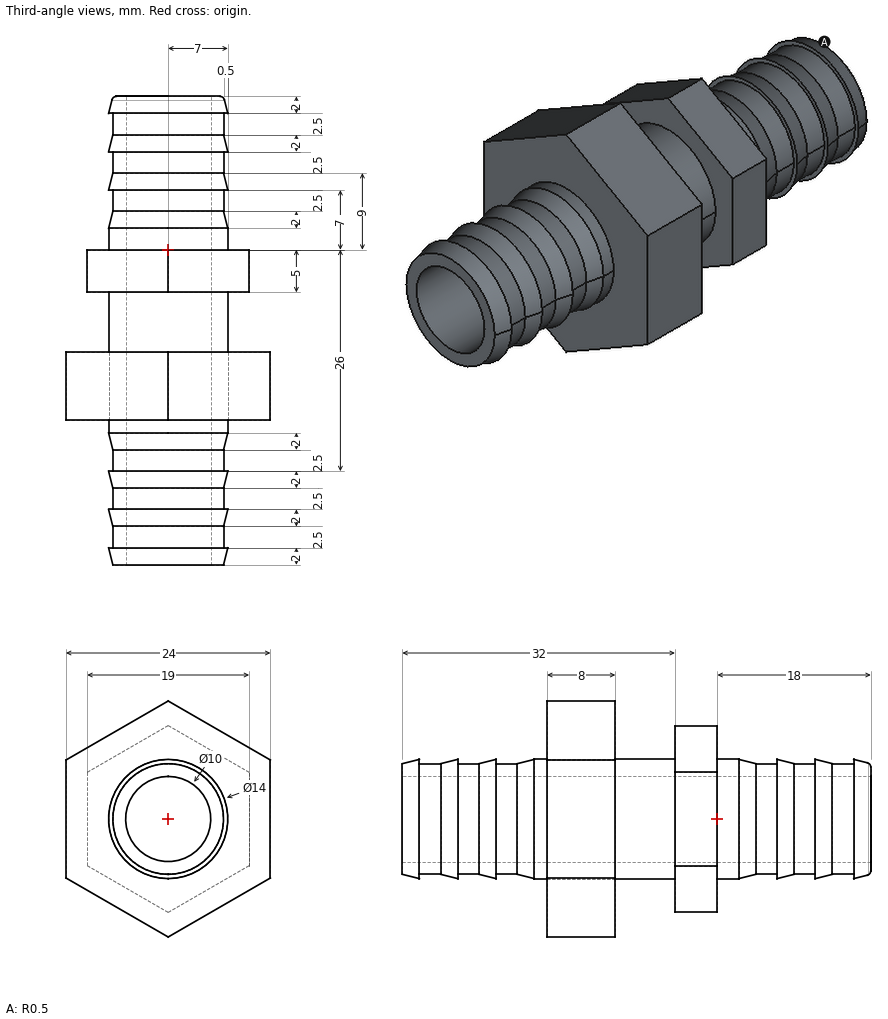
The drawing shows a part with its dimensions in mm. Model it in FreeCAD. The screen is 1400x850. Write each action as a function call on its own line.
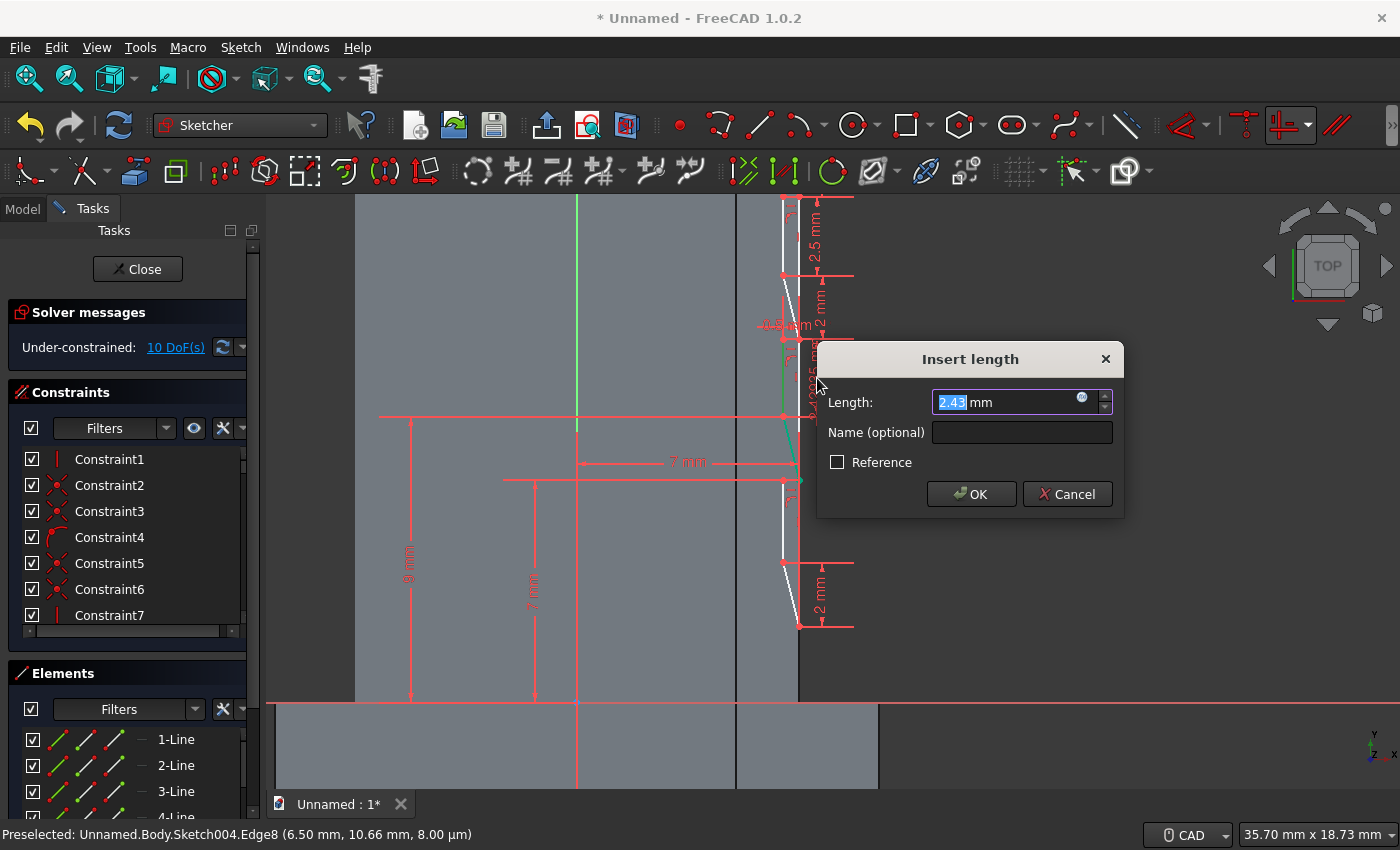
text(2.5)
key(Return)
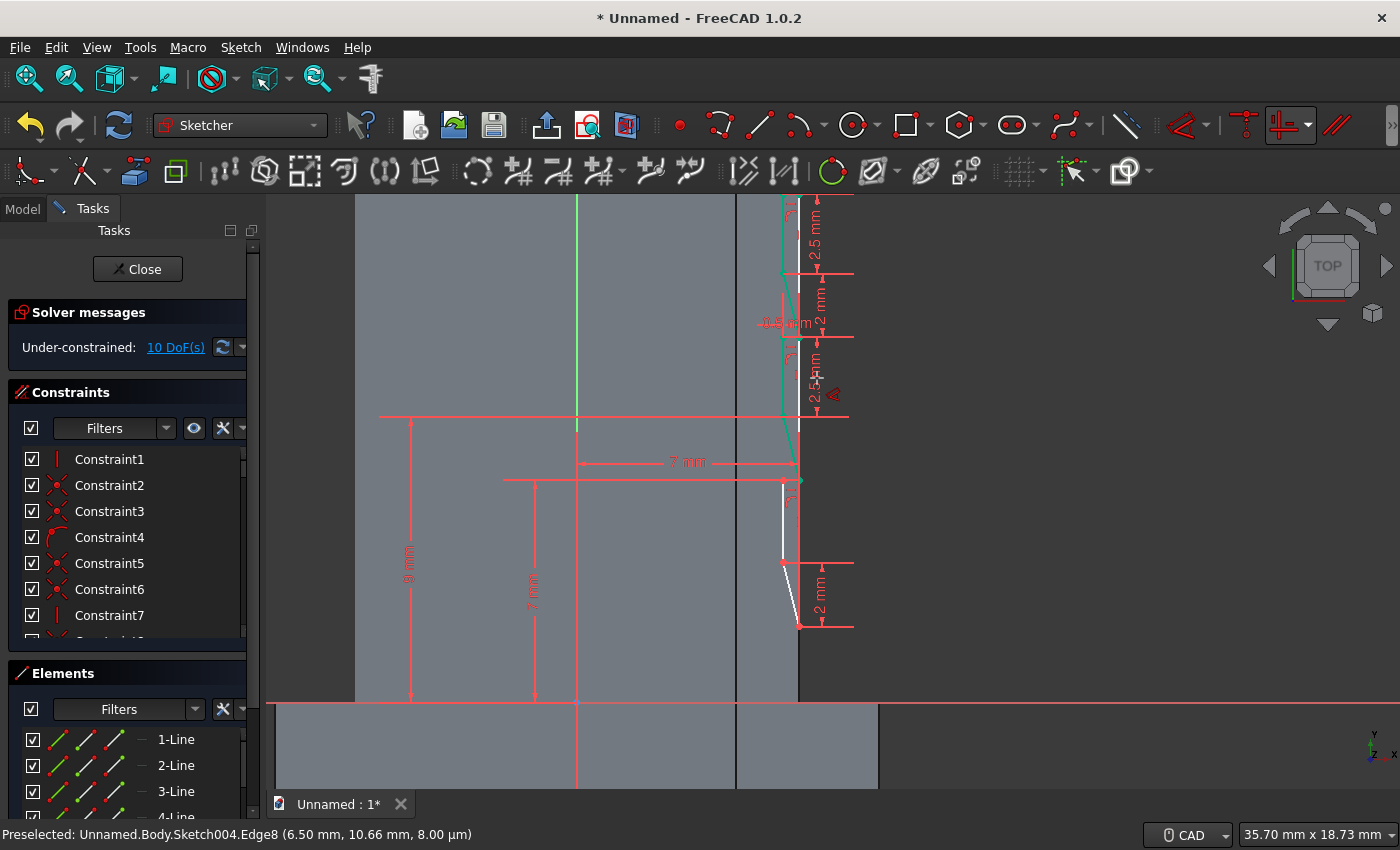
scroll(791, 480, up, 5)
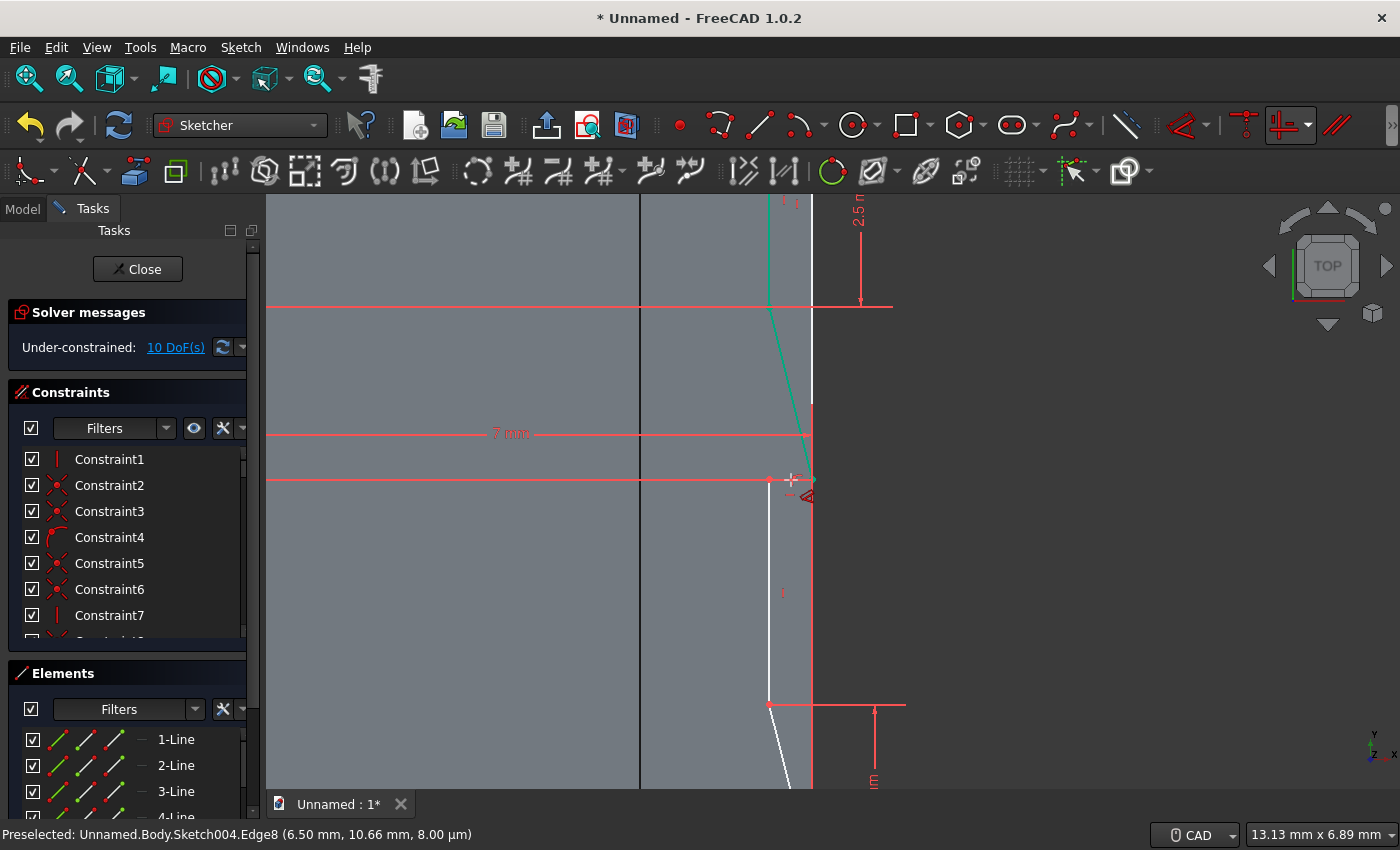
click(791, 480)
click(781, 446)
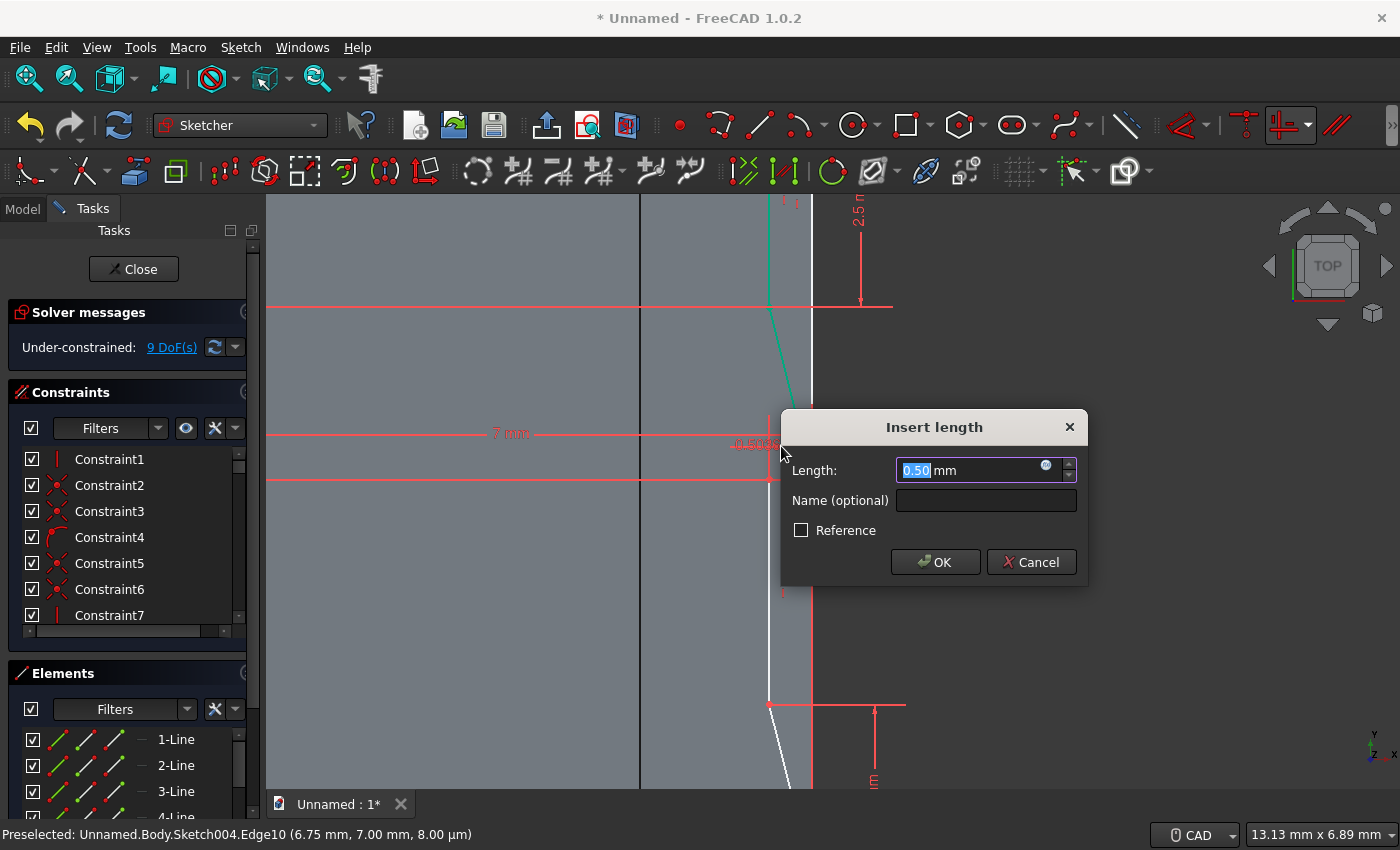
text(0.5)
key(Return)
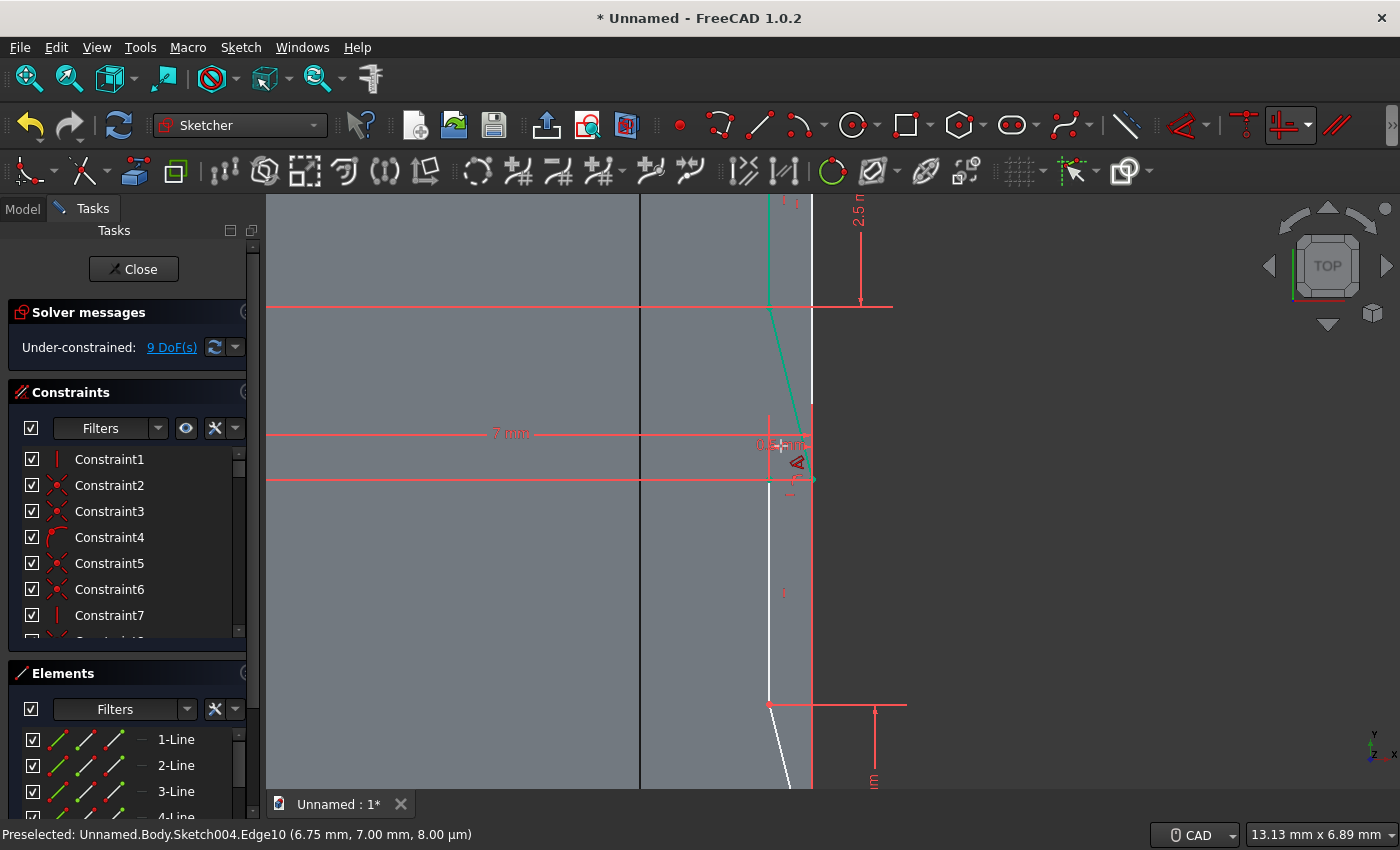
scroll(785, 378, down, 13)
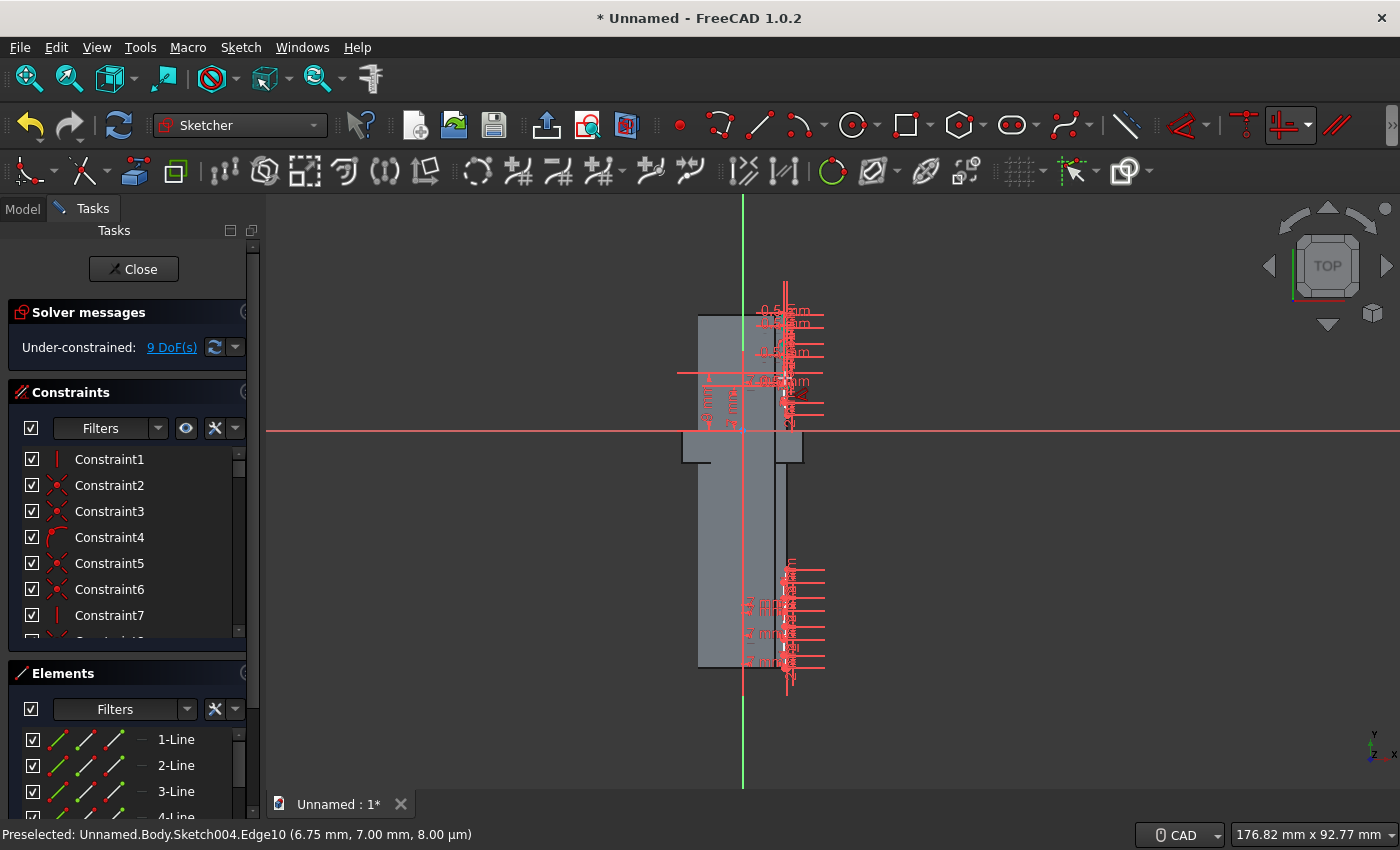
scroll(784, 391, up, 8)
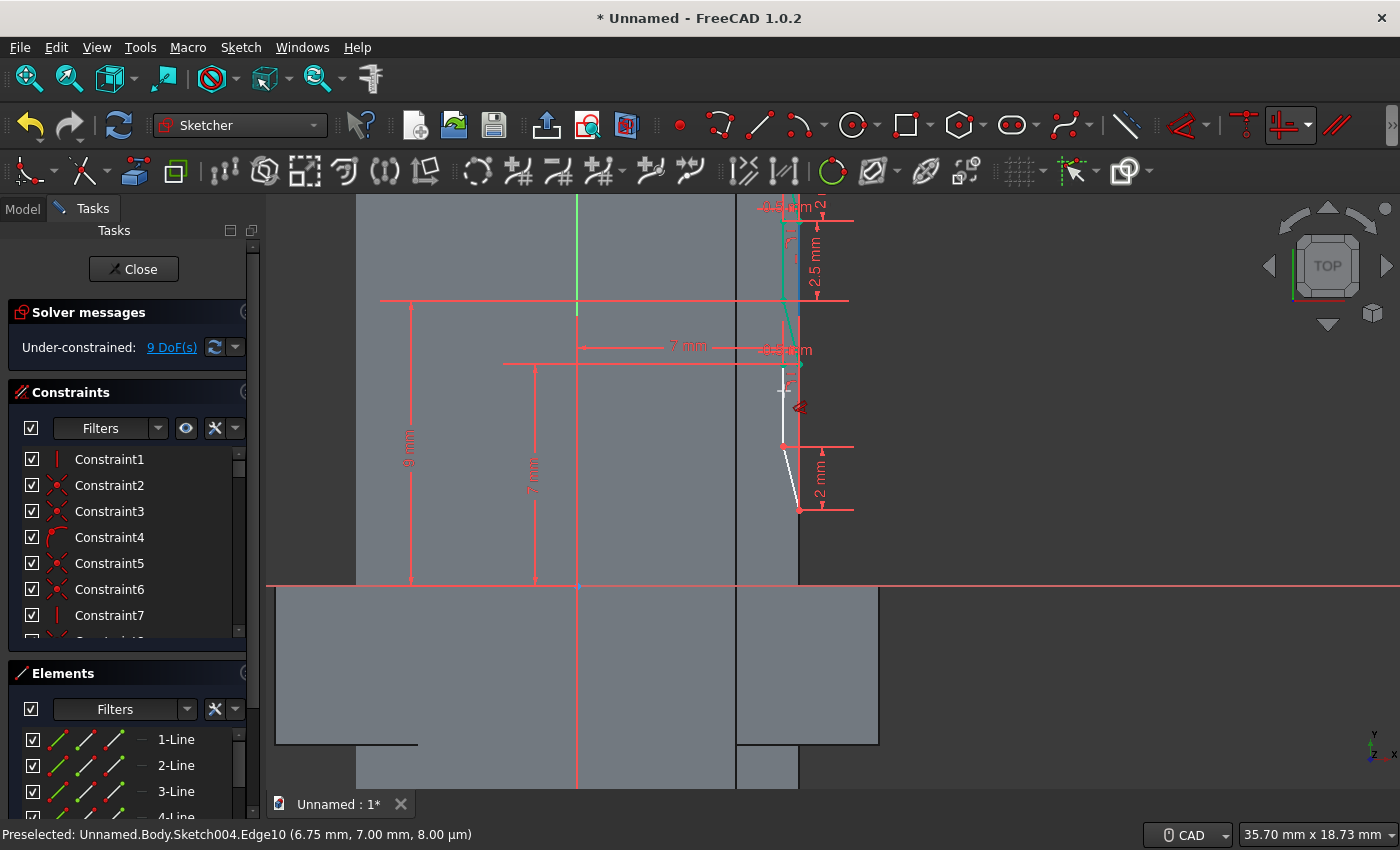
click(783, 389)
click(817, 406)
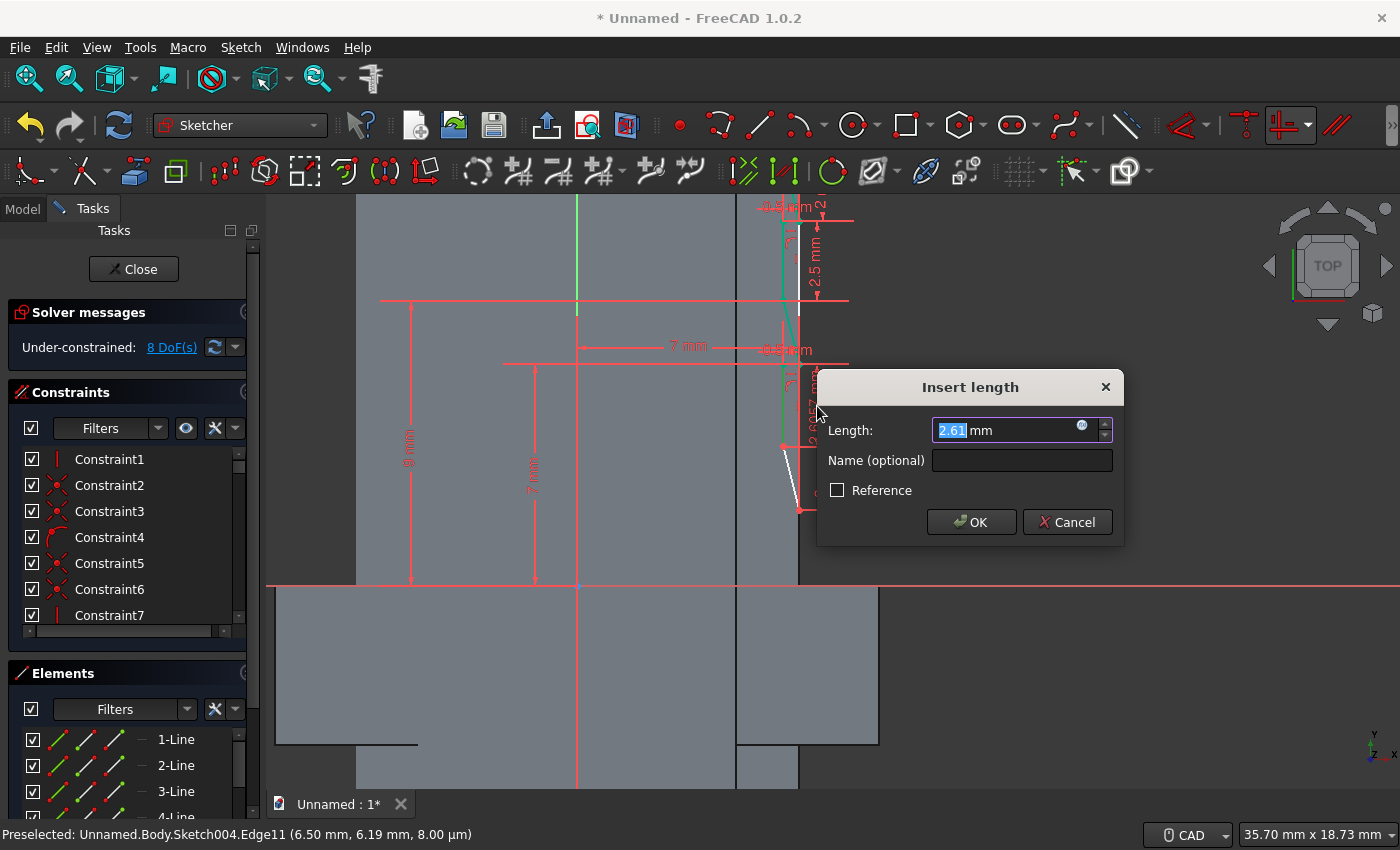
text(2.5)
key(Return)